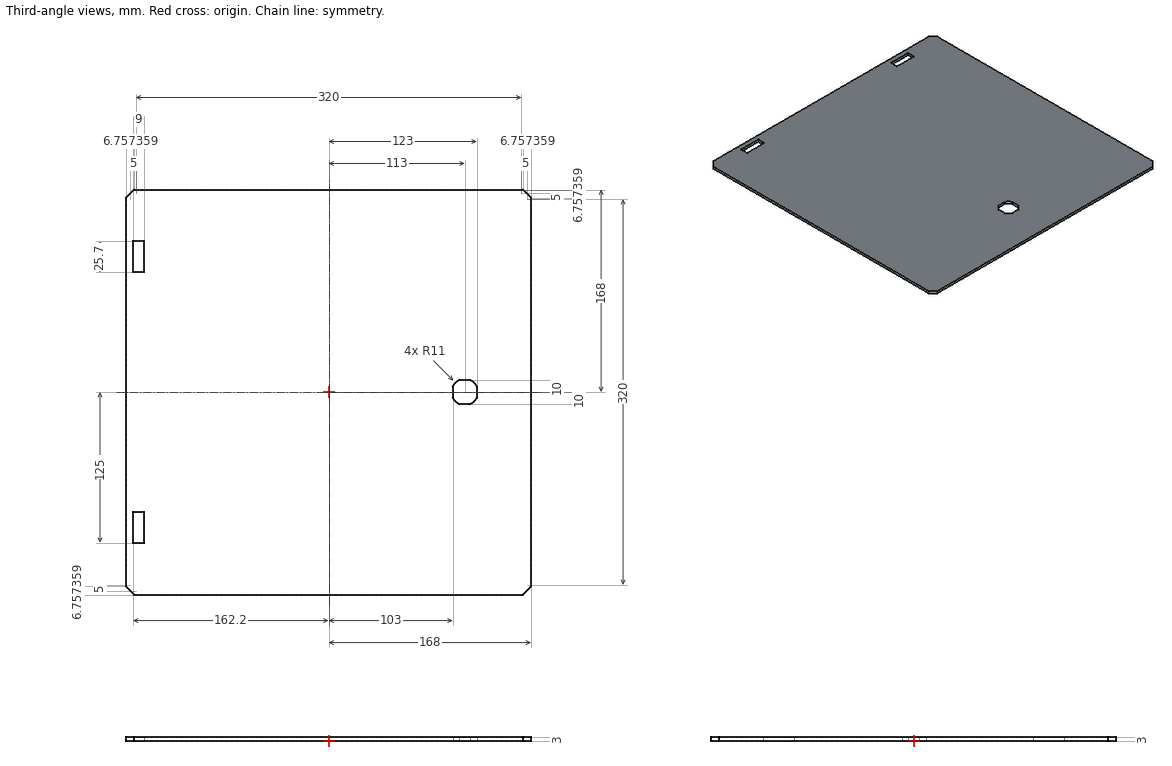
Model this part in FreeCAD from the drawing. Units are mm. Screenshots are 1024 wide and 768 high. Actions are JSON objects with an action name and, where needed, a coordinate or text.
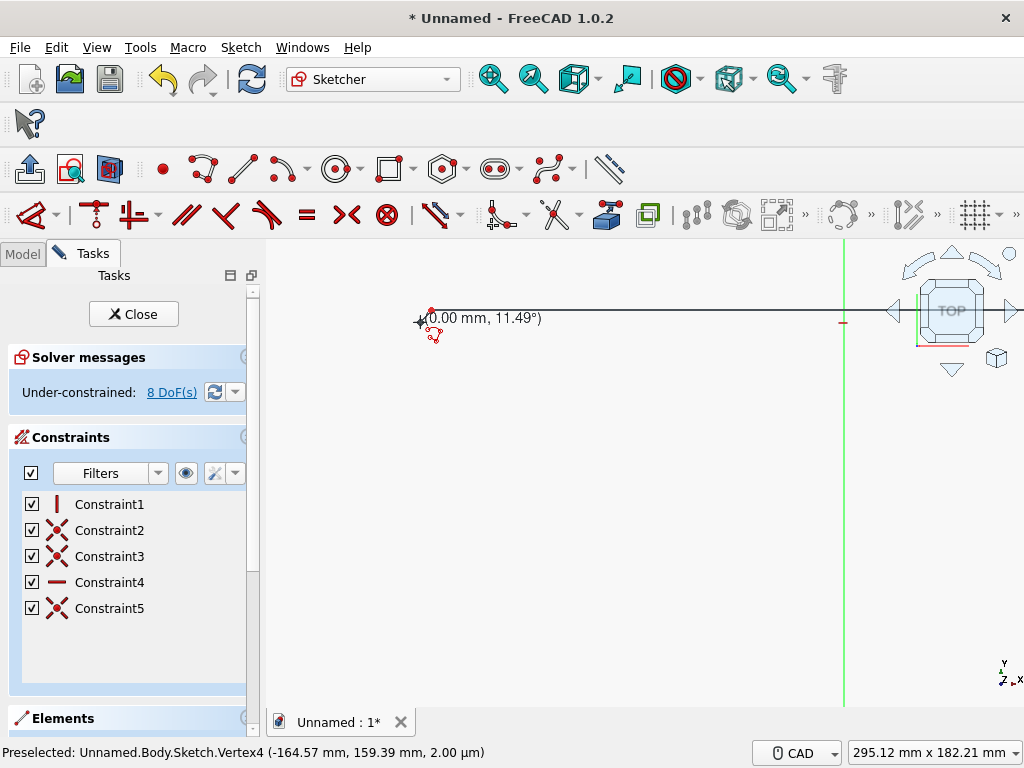
{"action": "scroll", "coordinate": [421, 322], "scroll_direction": "down", "scroll_amount": 5}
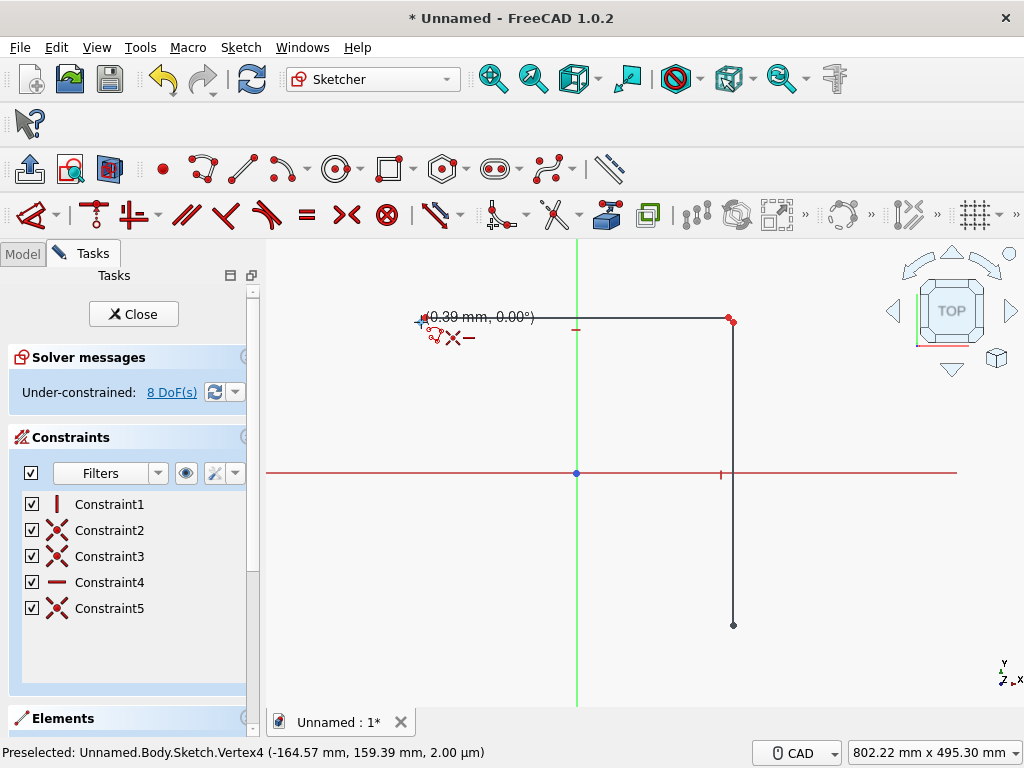
{"action": "left_click", "coordinate": [421, 625]}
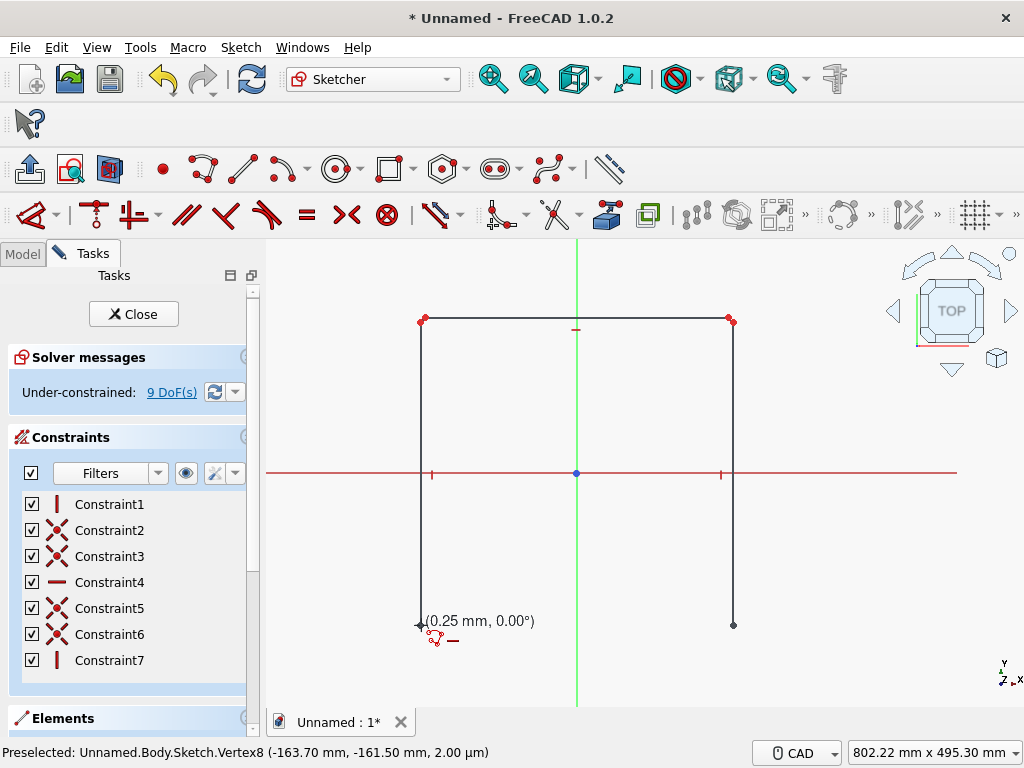
{"action": "scroll", "coordinate": [425, 629], "scroll_direction": "up", "scroll_amount": 5}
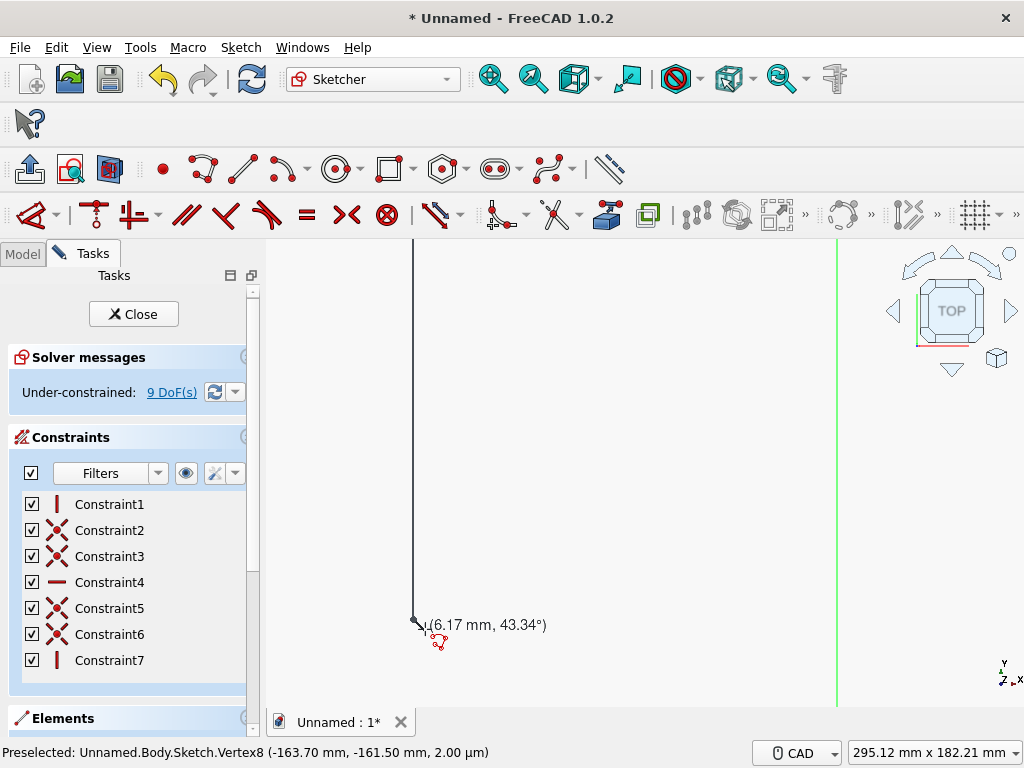
{"action": "left_click", "coordinate": [426, 628]}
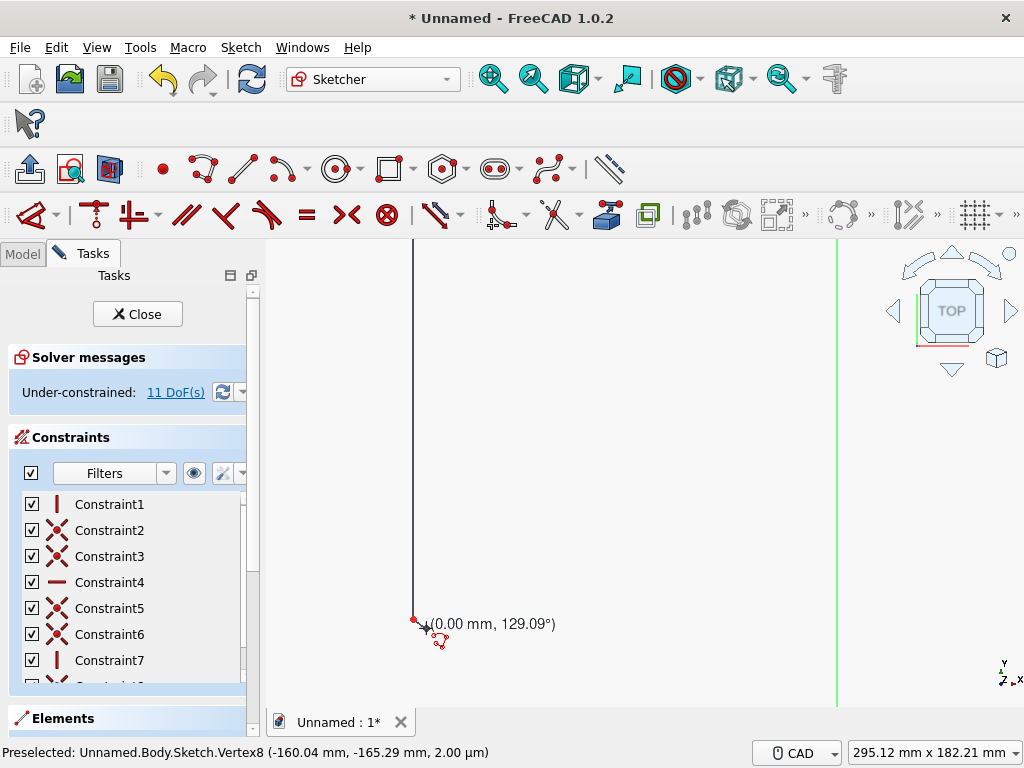
{"action": "scroll", "coordinate": [425, 629], "scroll_direction": "down", "scroll_amount": 5}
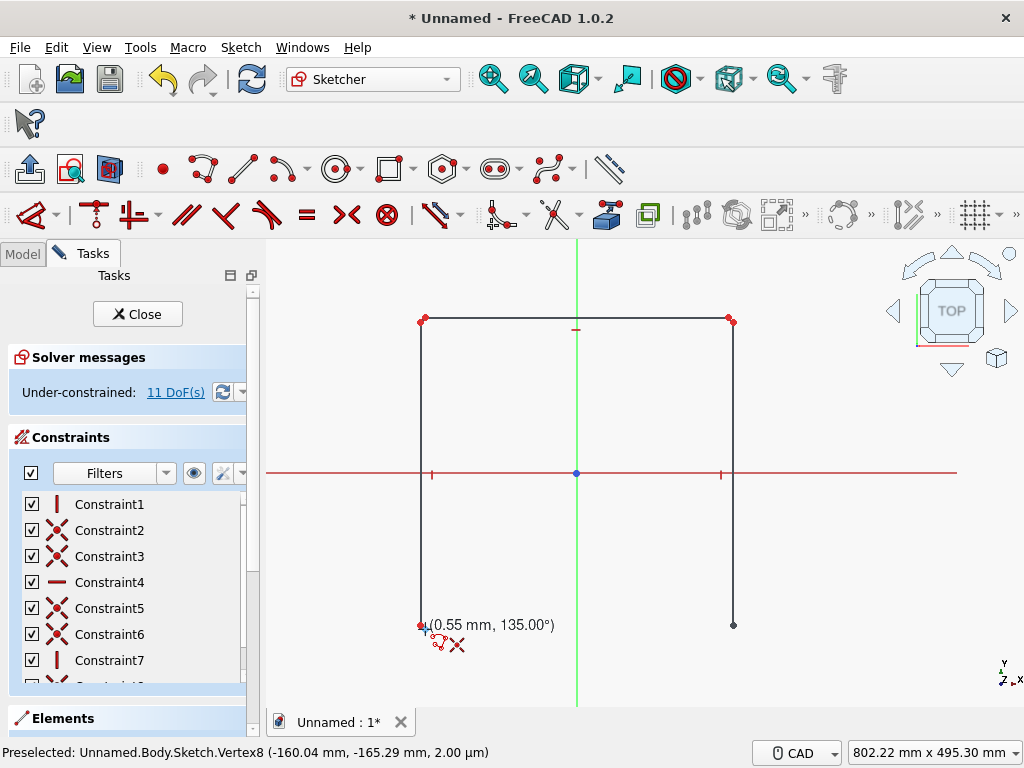
{"action": "scroll", "coordinate": [728, 629], "scroll_direction": "up", "scroll_amount": 5}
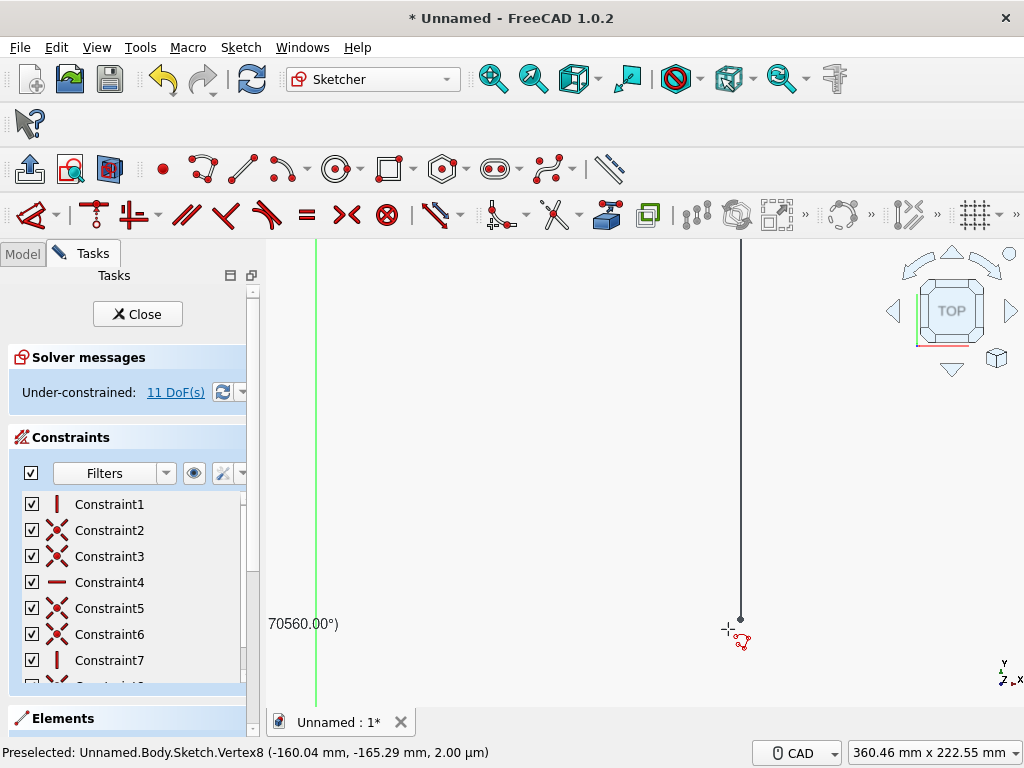
{"action": "left_click", "coordinate": [727, 628]}
{"action": "left_click", "coordinate": [741, 619]}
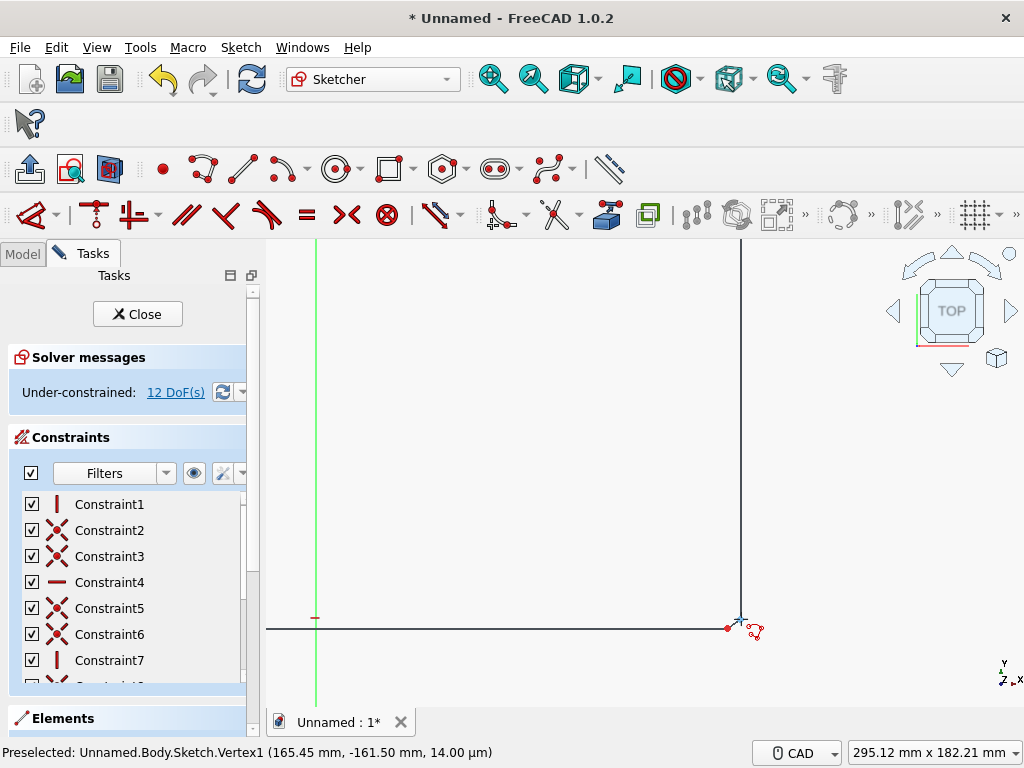
{"action": "left_click", "coordinate": [390, 170]}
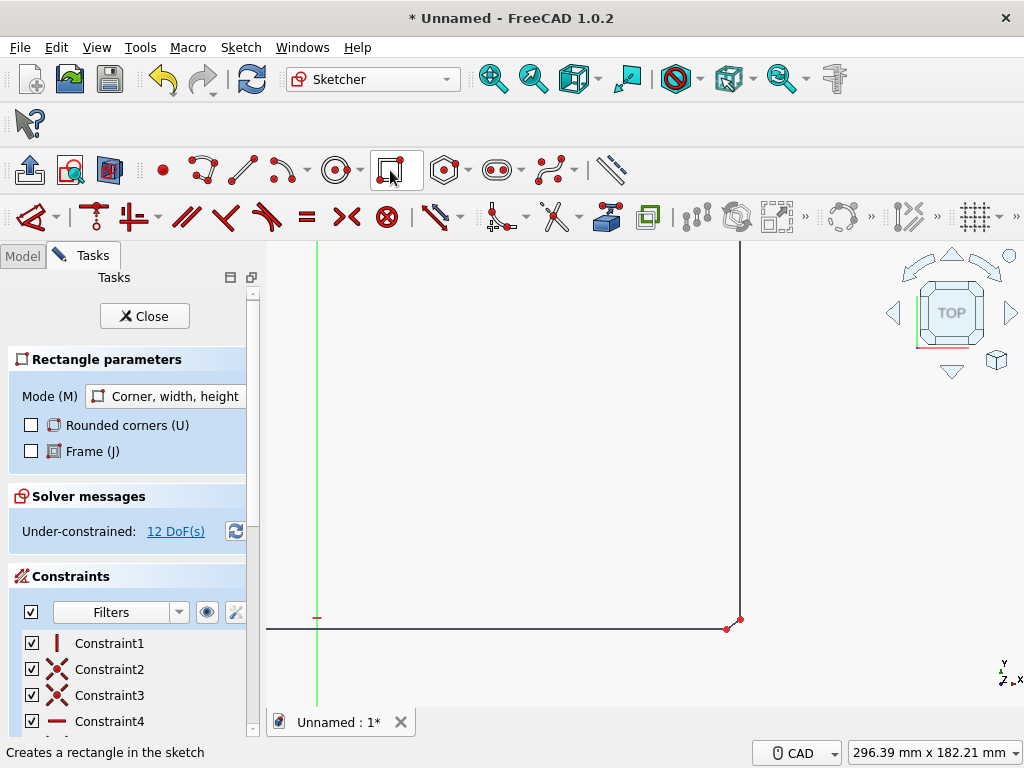
{"action": "scroll", "coordinate": [728, 630], "scroll_direction": "down", "scroll_amount": 5}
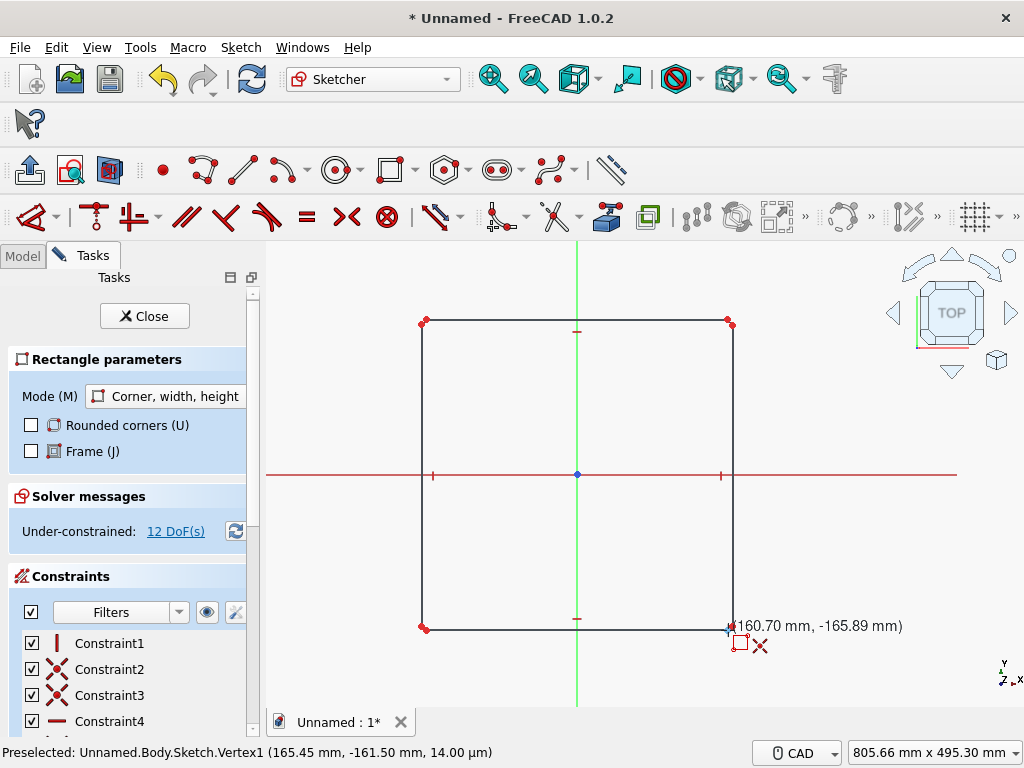
{"action": "scroll", "coordinate": [425, 568], "scroll_direction": "up", "scroll_amount": 9}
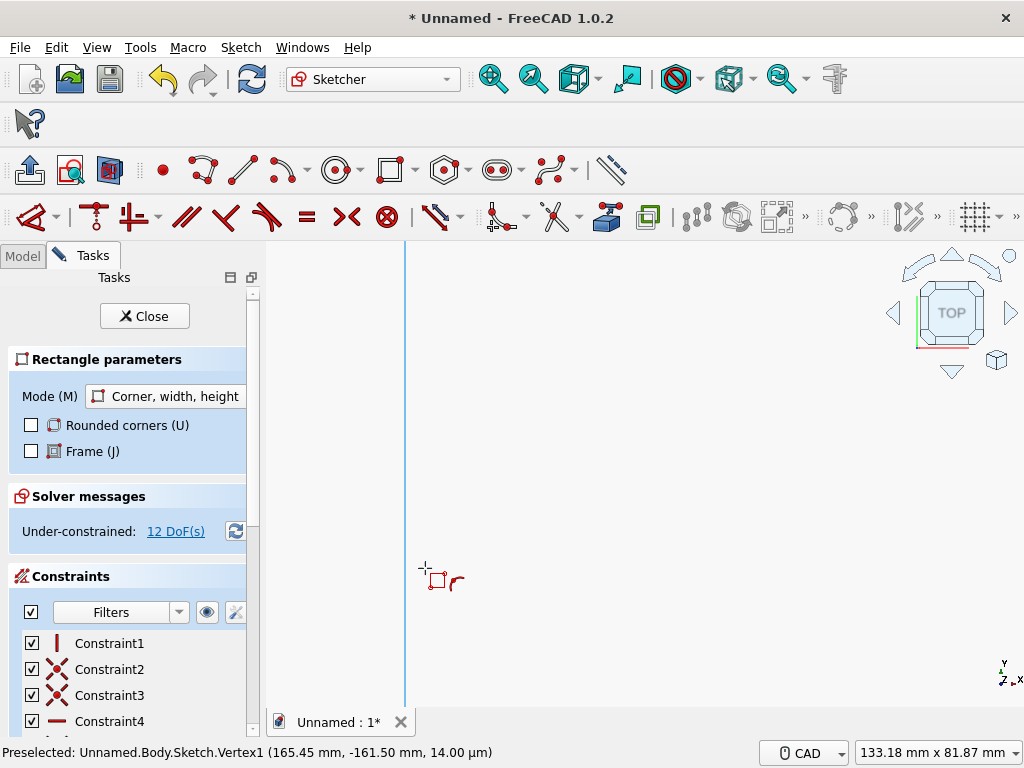
{"action": "left_click", "coordinate": [421, 566]}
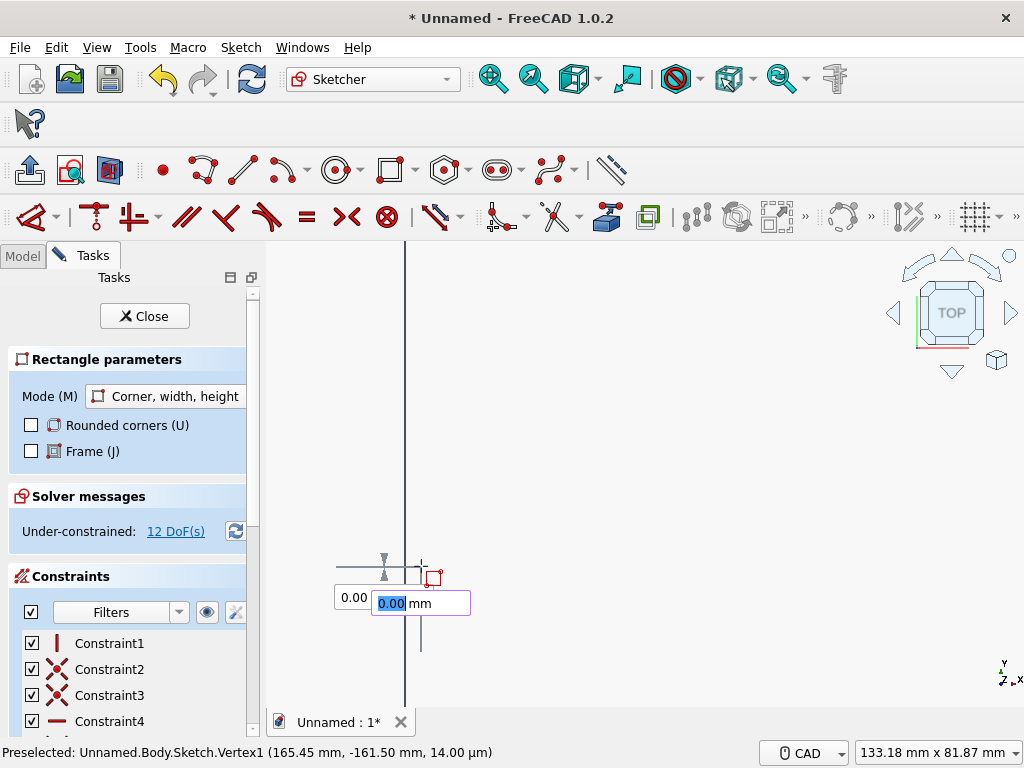
{"action": "scroll", "coordinate": [424, 568], "scroll_direction": "down", "scroll_amount": 9}